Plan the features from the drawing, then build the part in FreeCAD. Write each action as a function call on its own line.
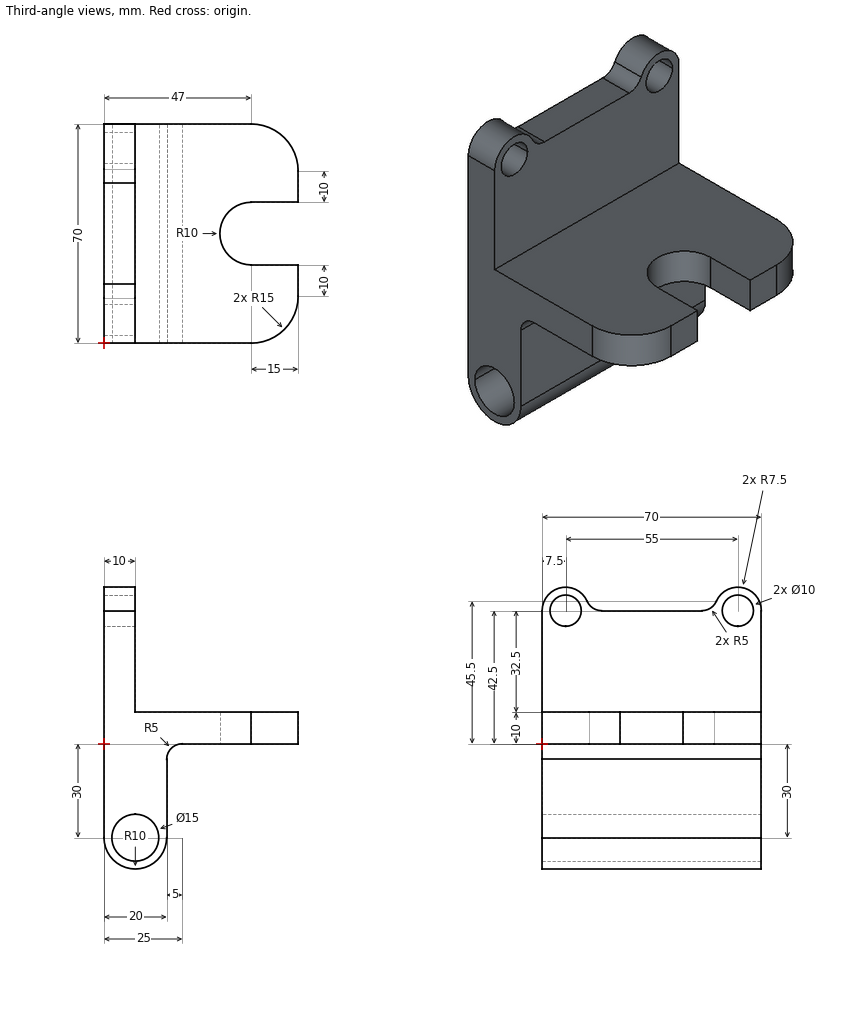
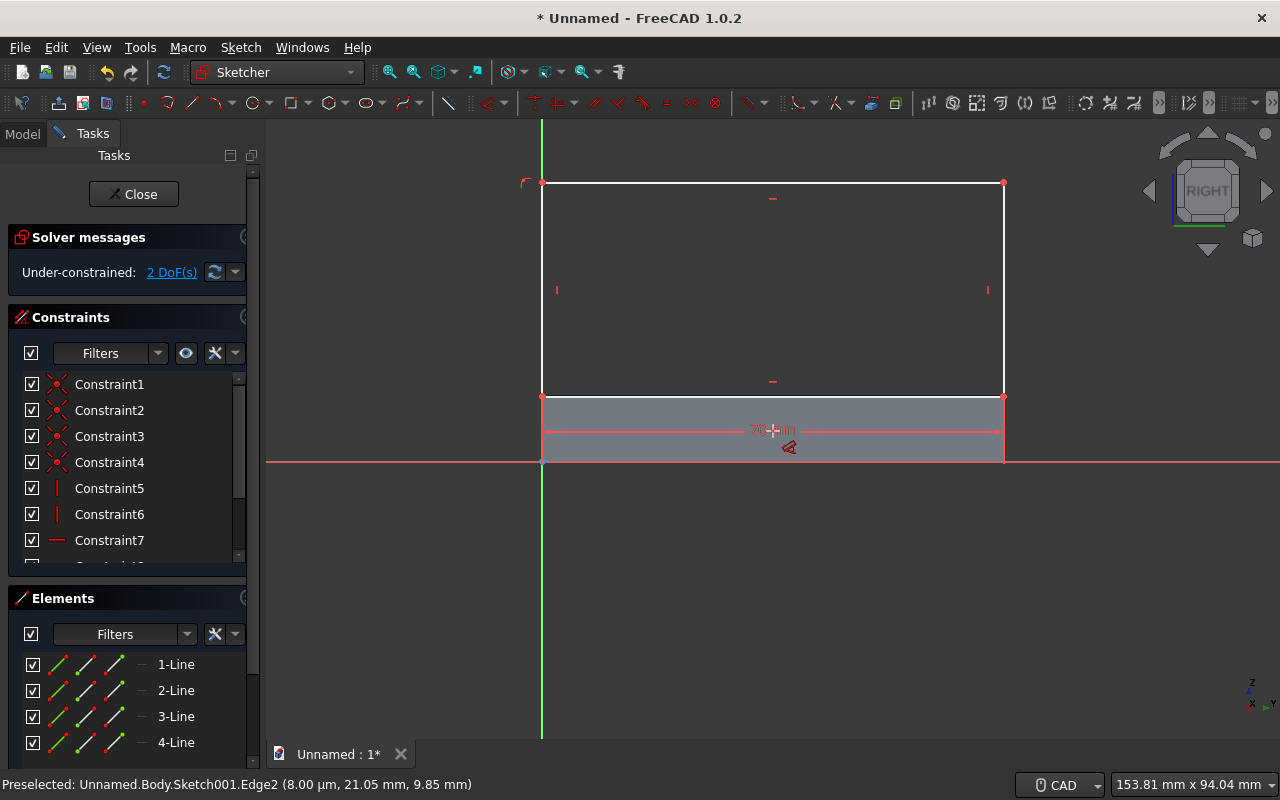
click(542, 397)
click(508, 429)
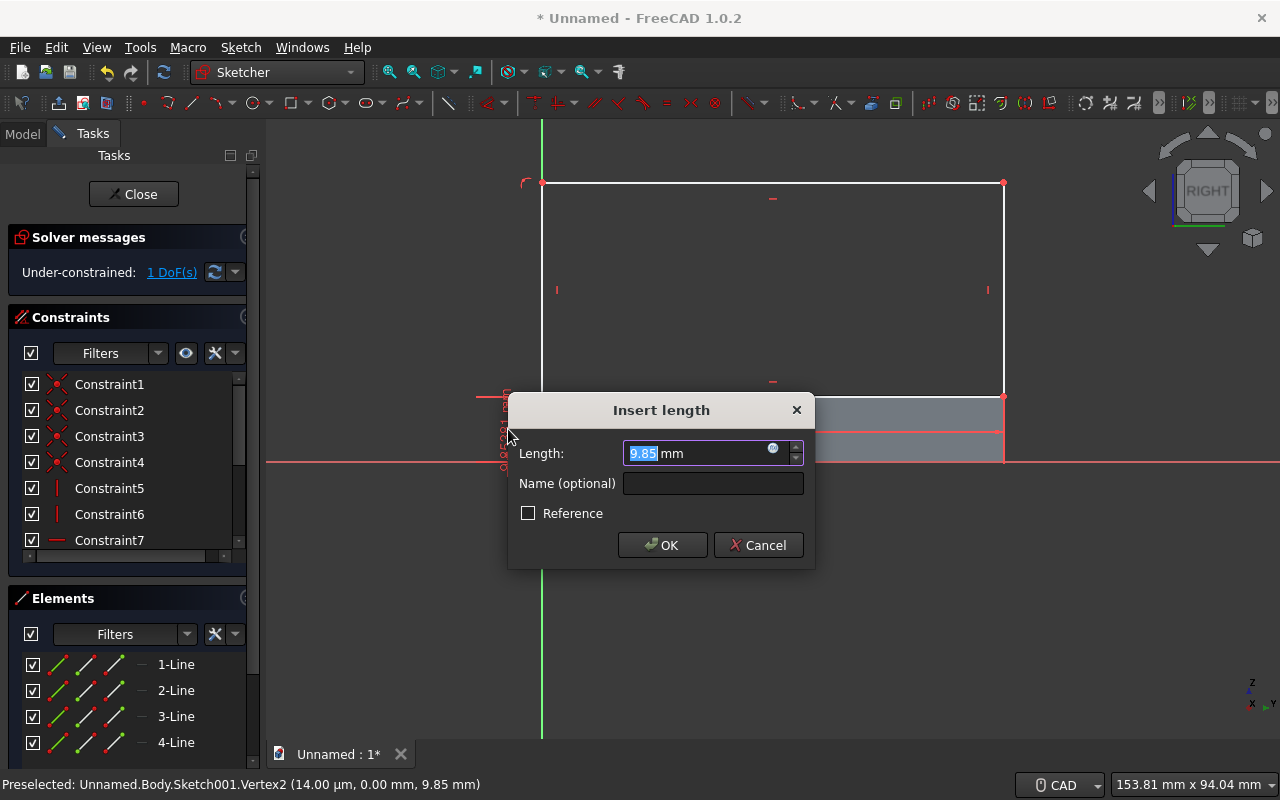
text(10)
key(Return)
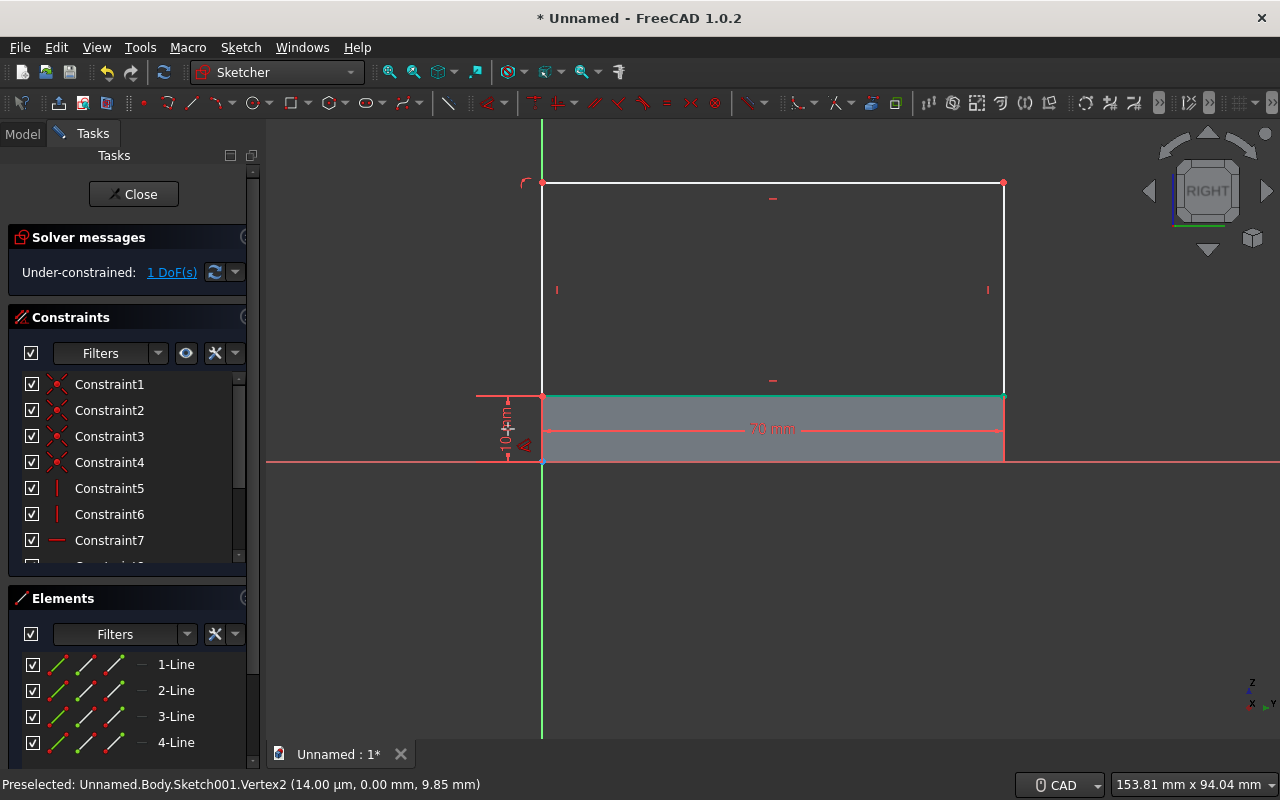
click(542, 247)
click(508, 290)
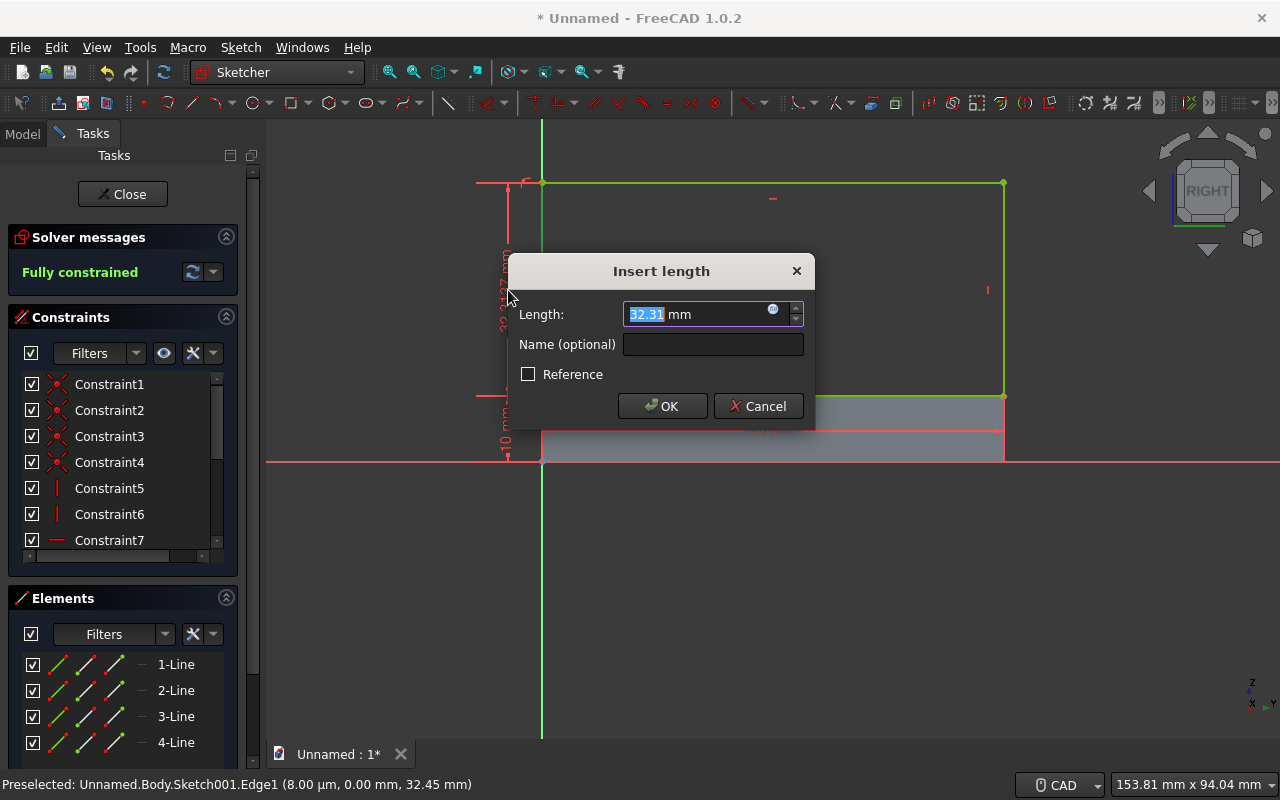
text(32.5)
key(Return)
key(Escape)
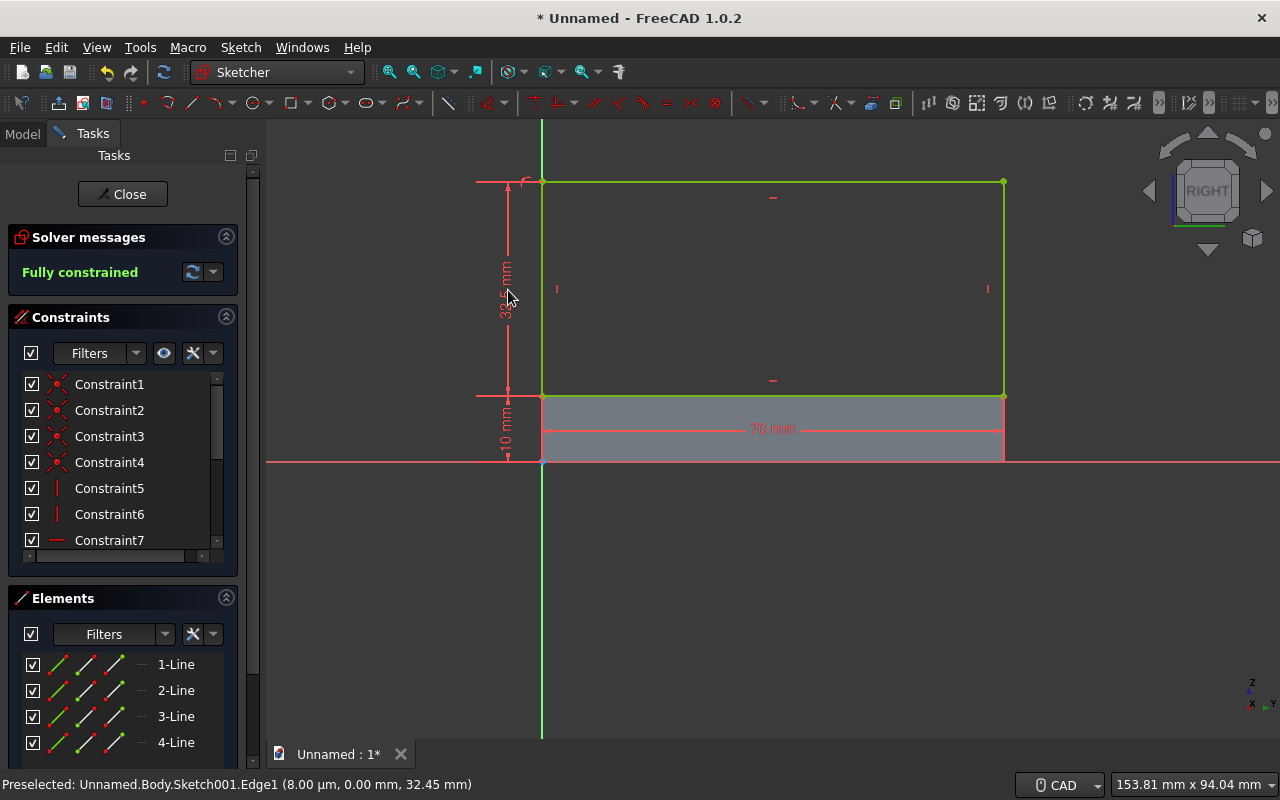
click(123, 194)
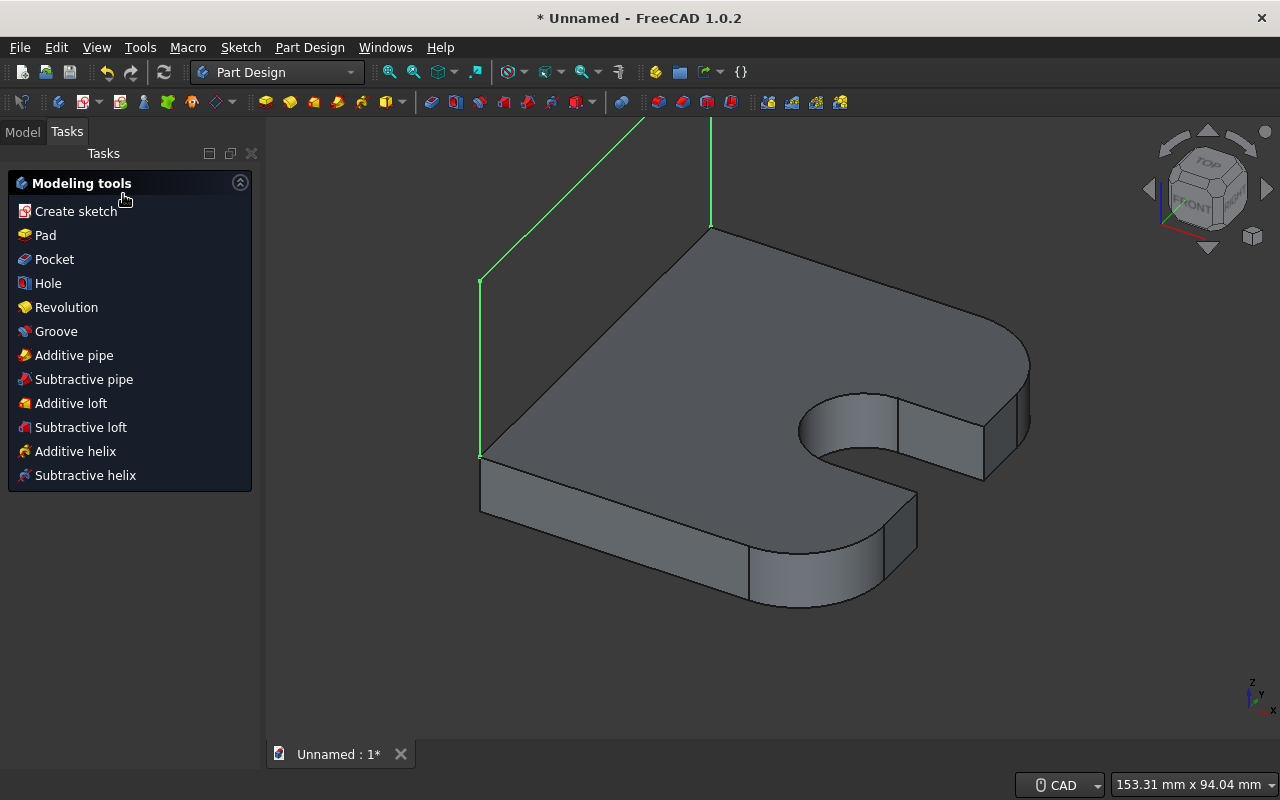
click(266, 102)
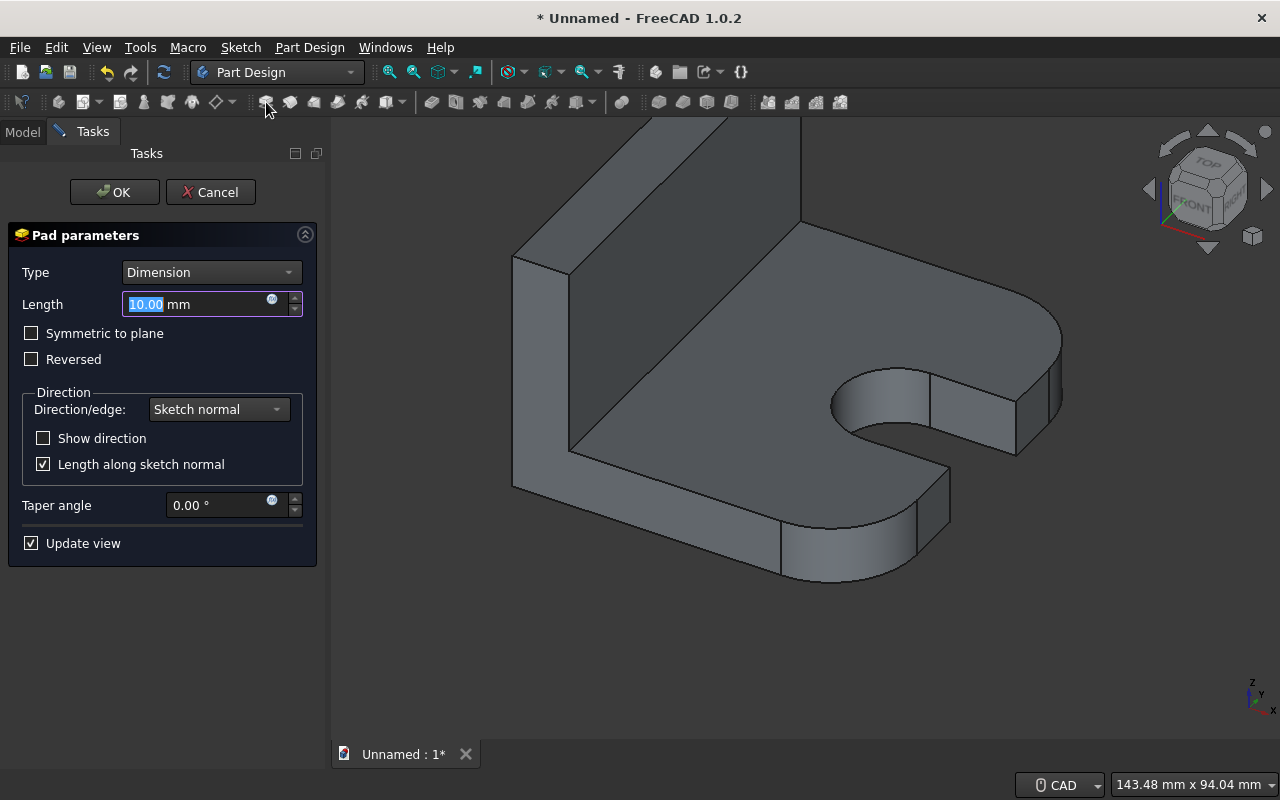
text(10)
key(Tab)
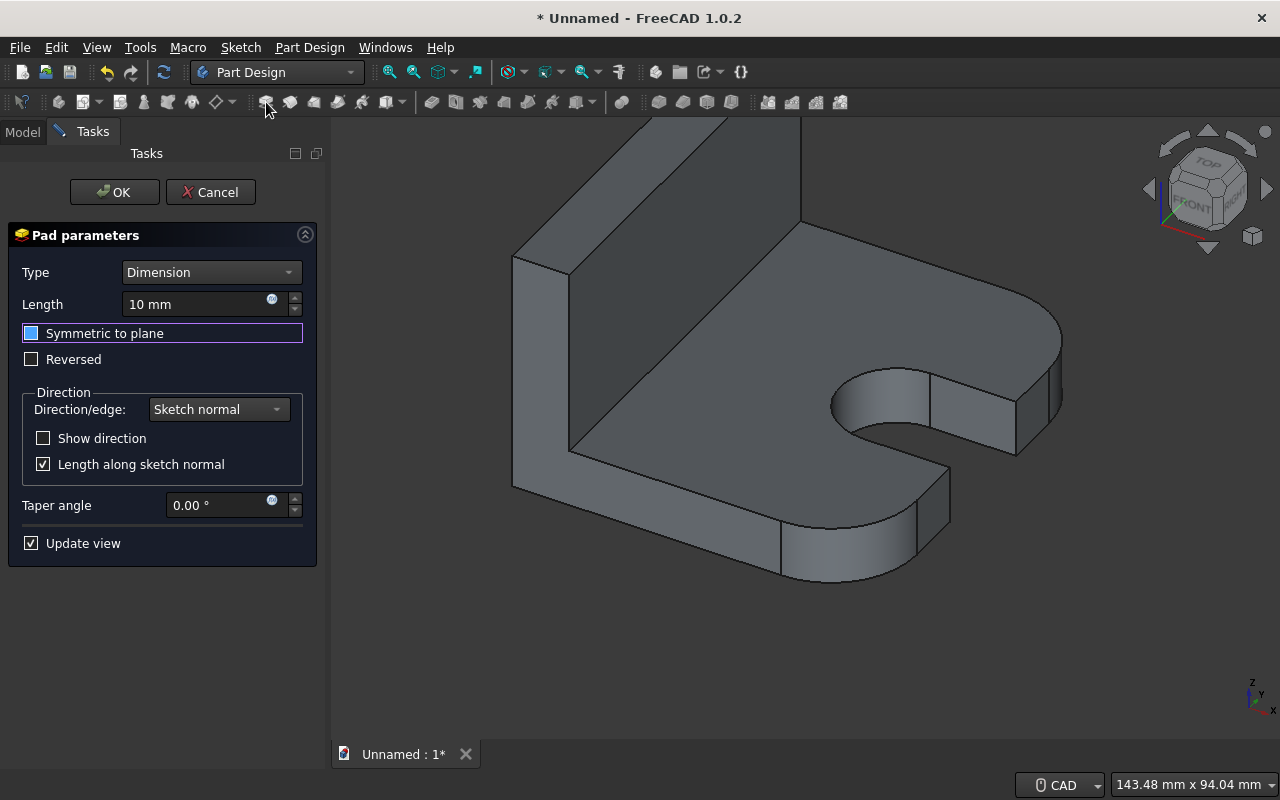
click(115, 192)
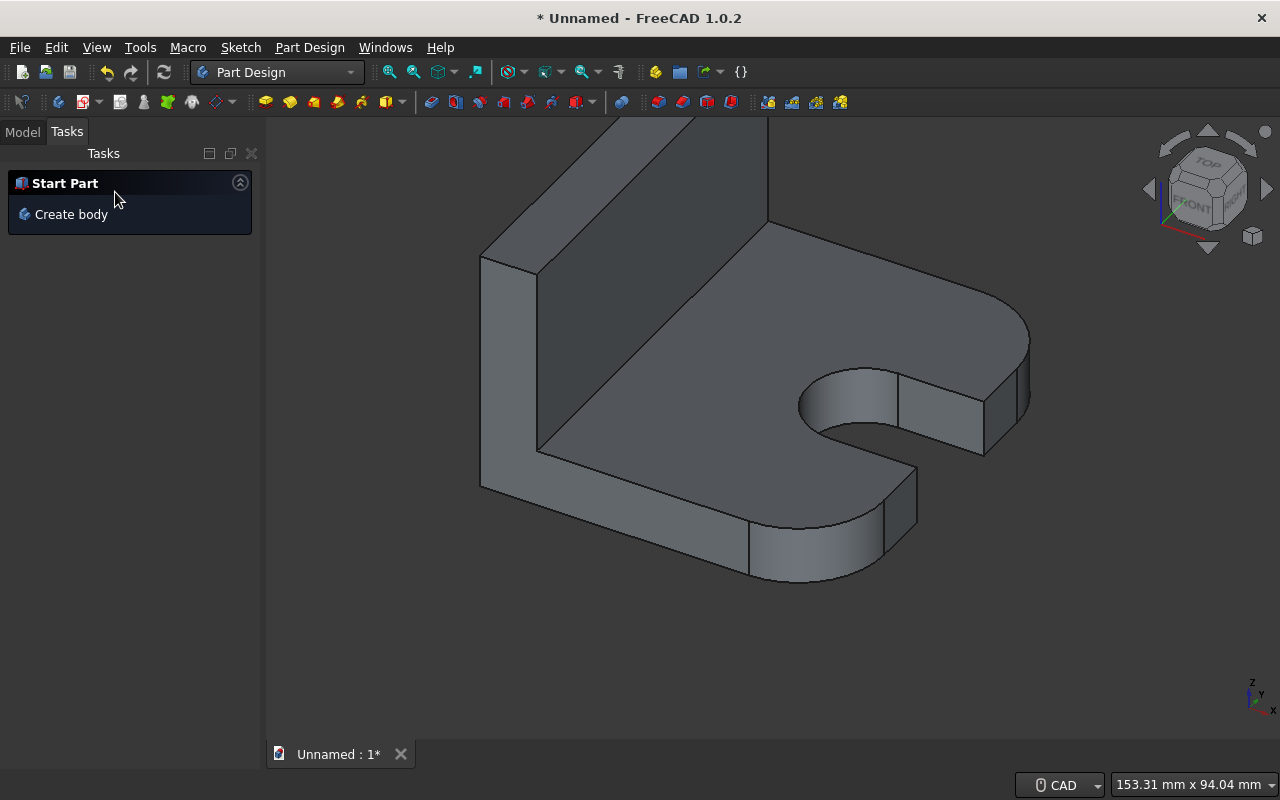
click(390, 72)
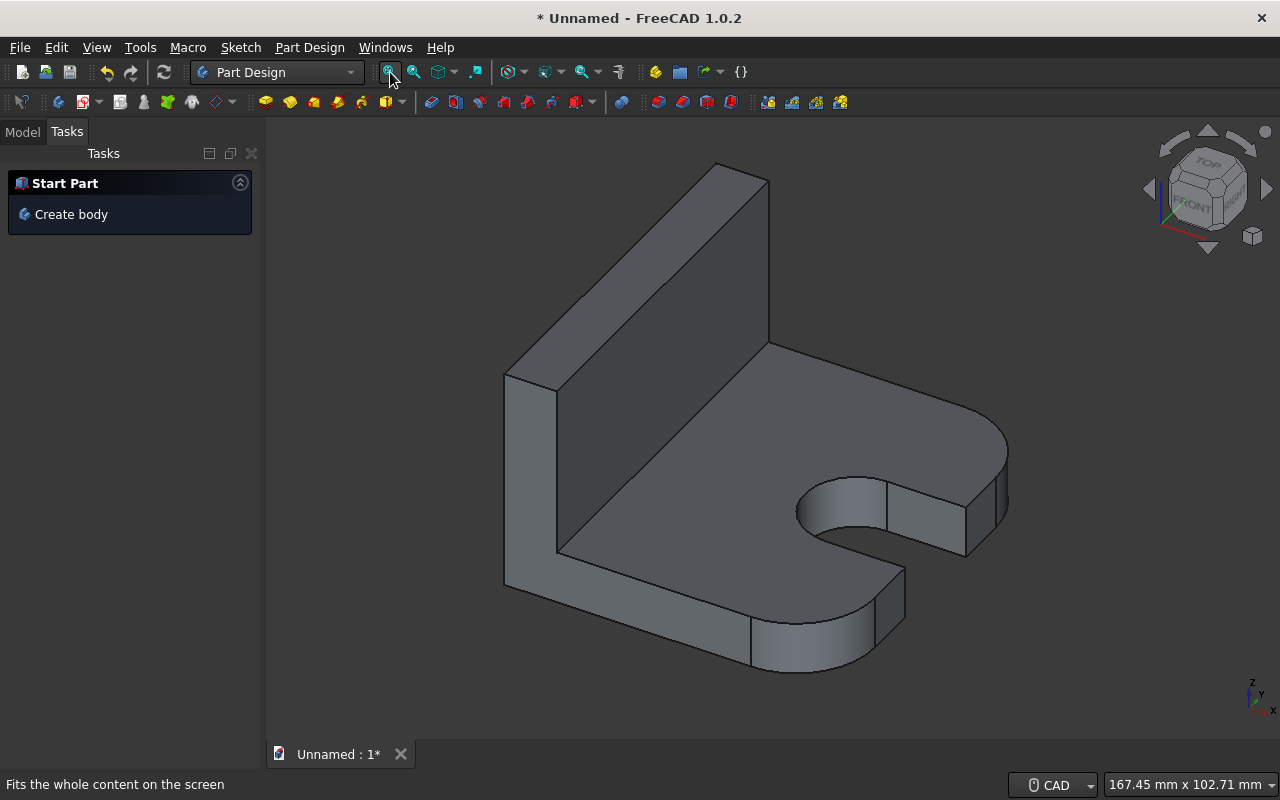
click(693, 336)